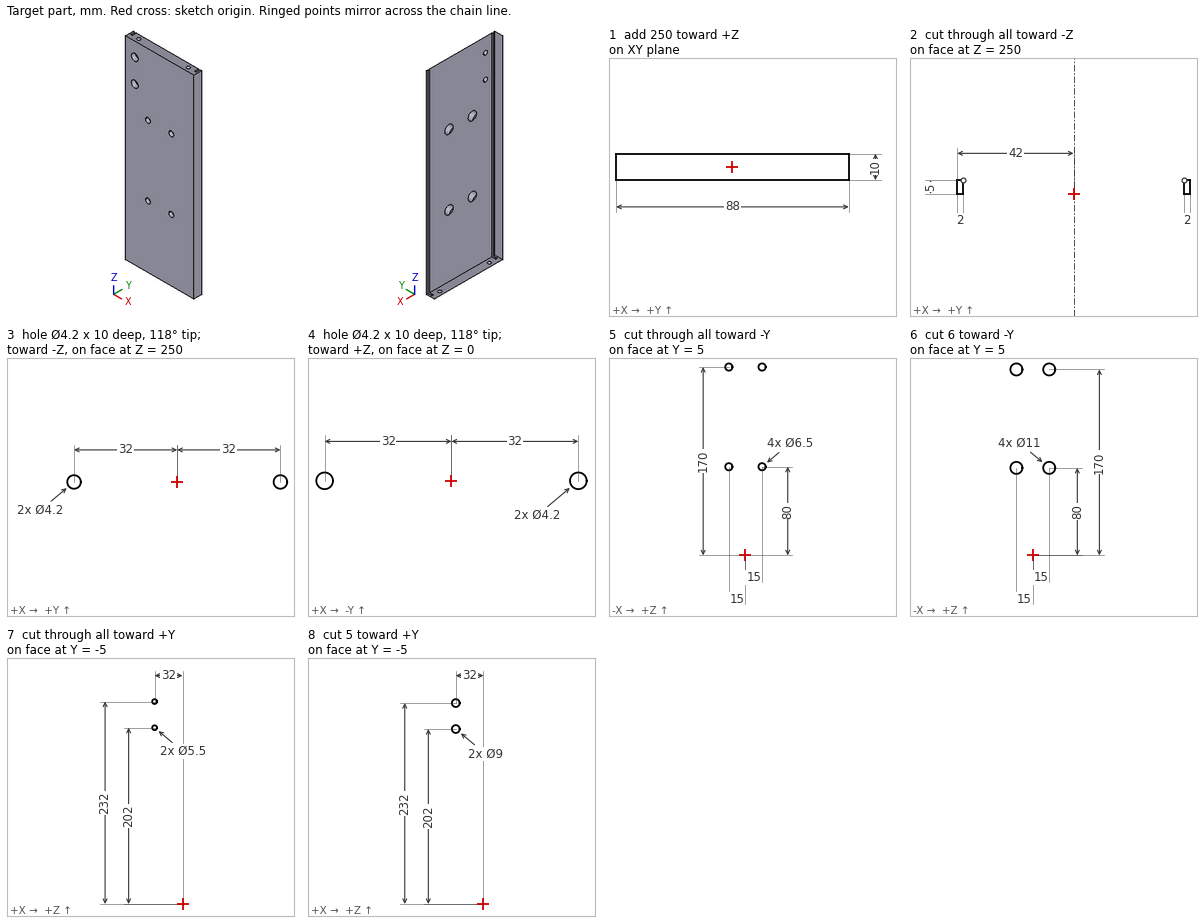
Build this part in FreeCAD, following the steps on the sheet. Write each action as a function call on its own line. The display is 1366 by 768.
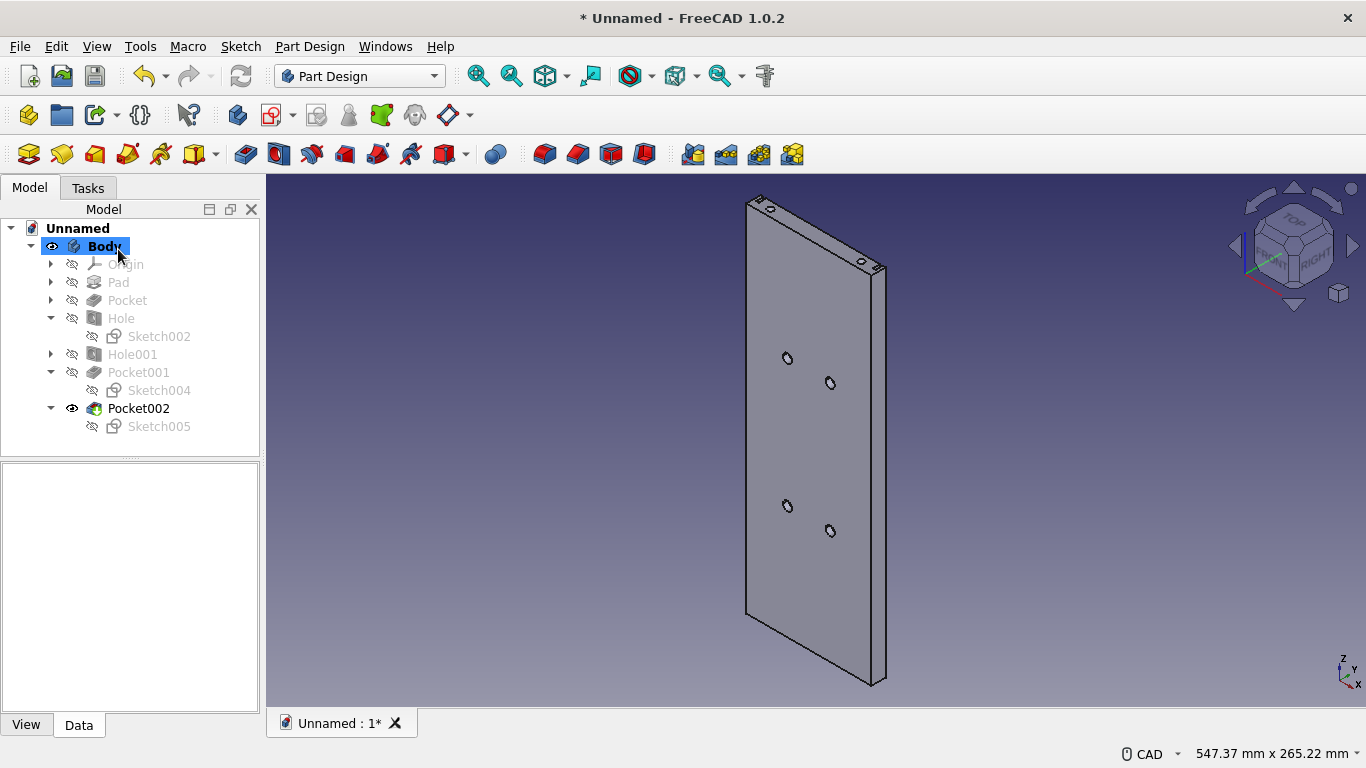
click(809, 444)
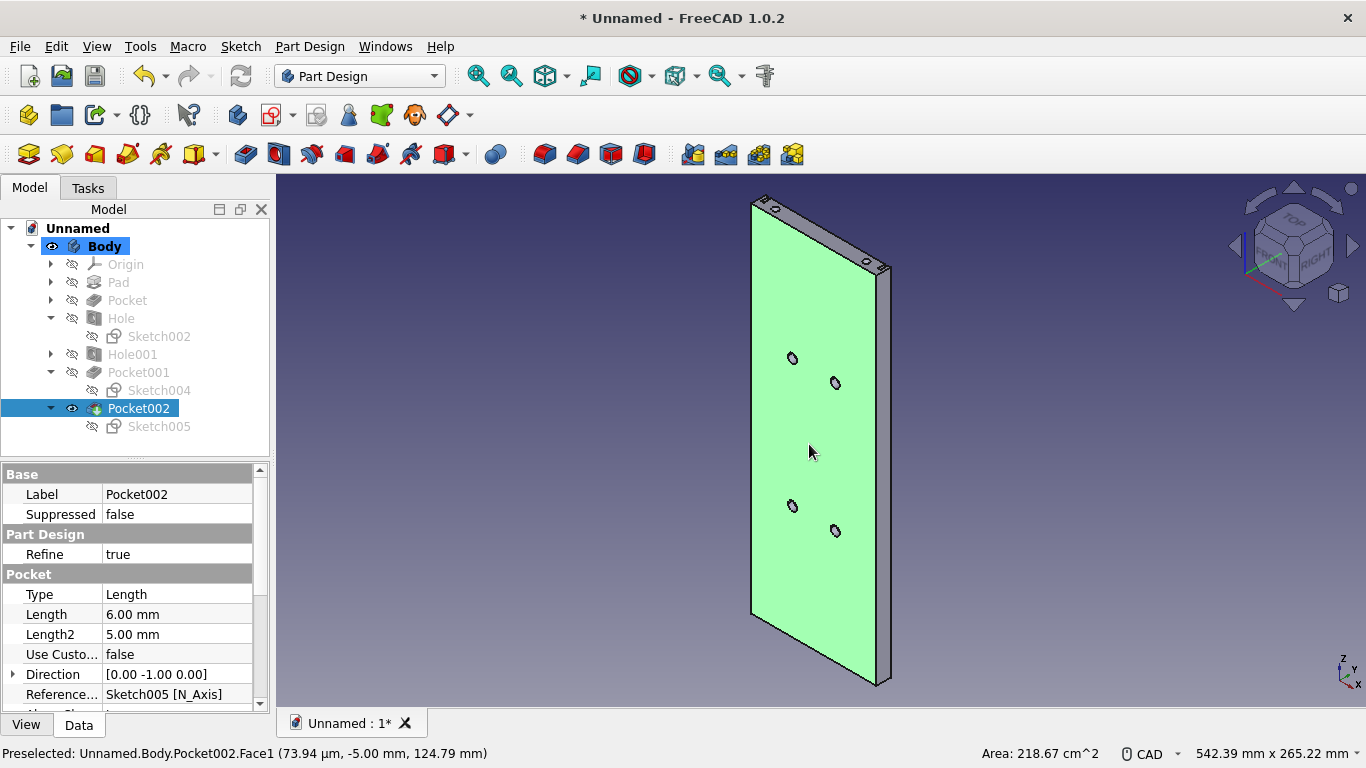
click(270, 116)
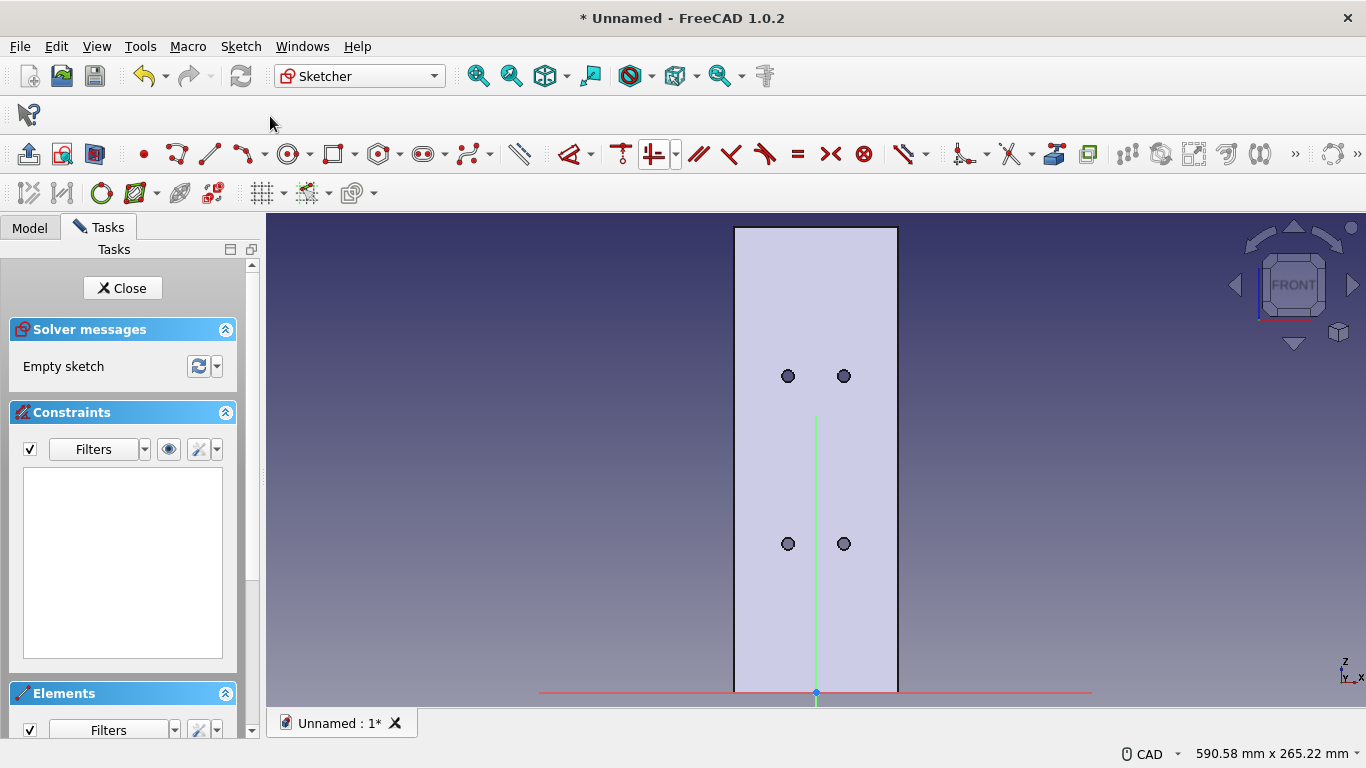
scroll(759, 245, up, 8)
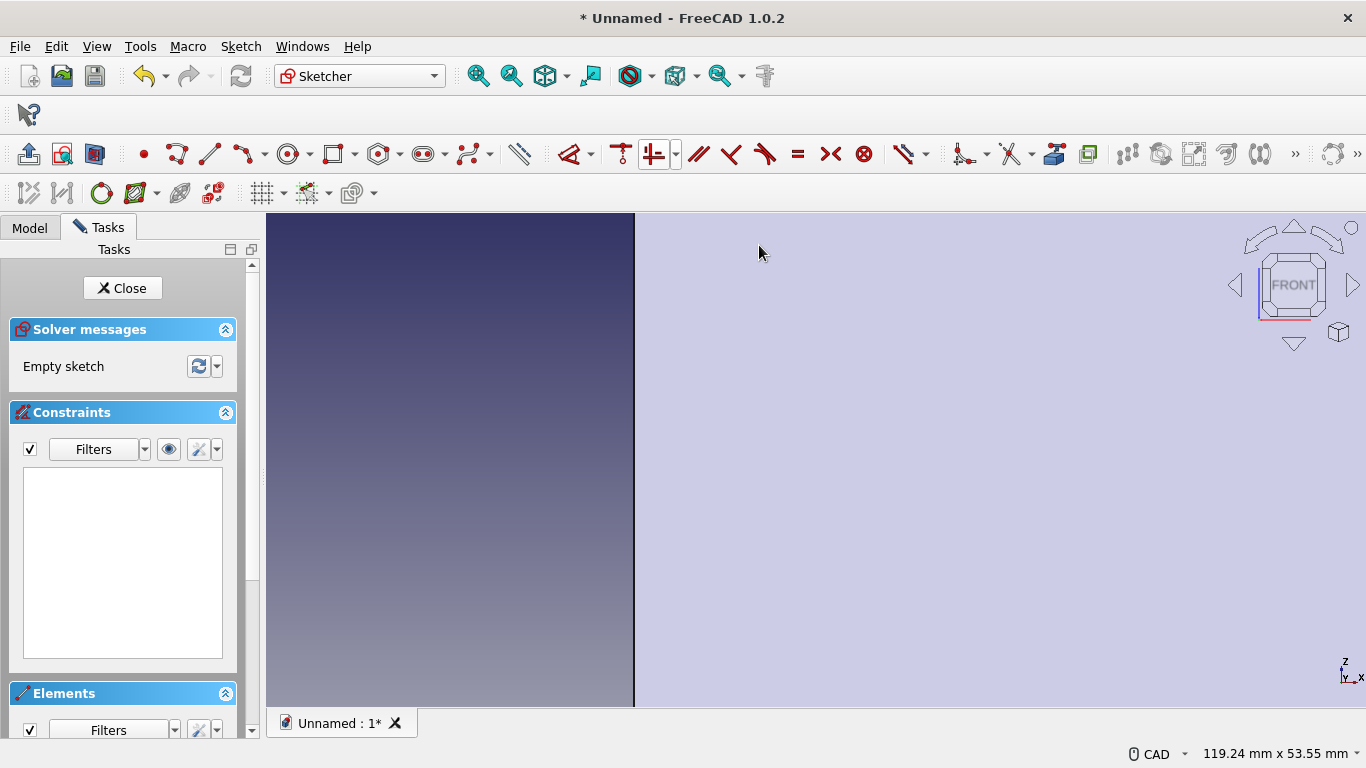
click(288, 154)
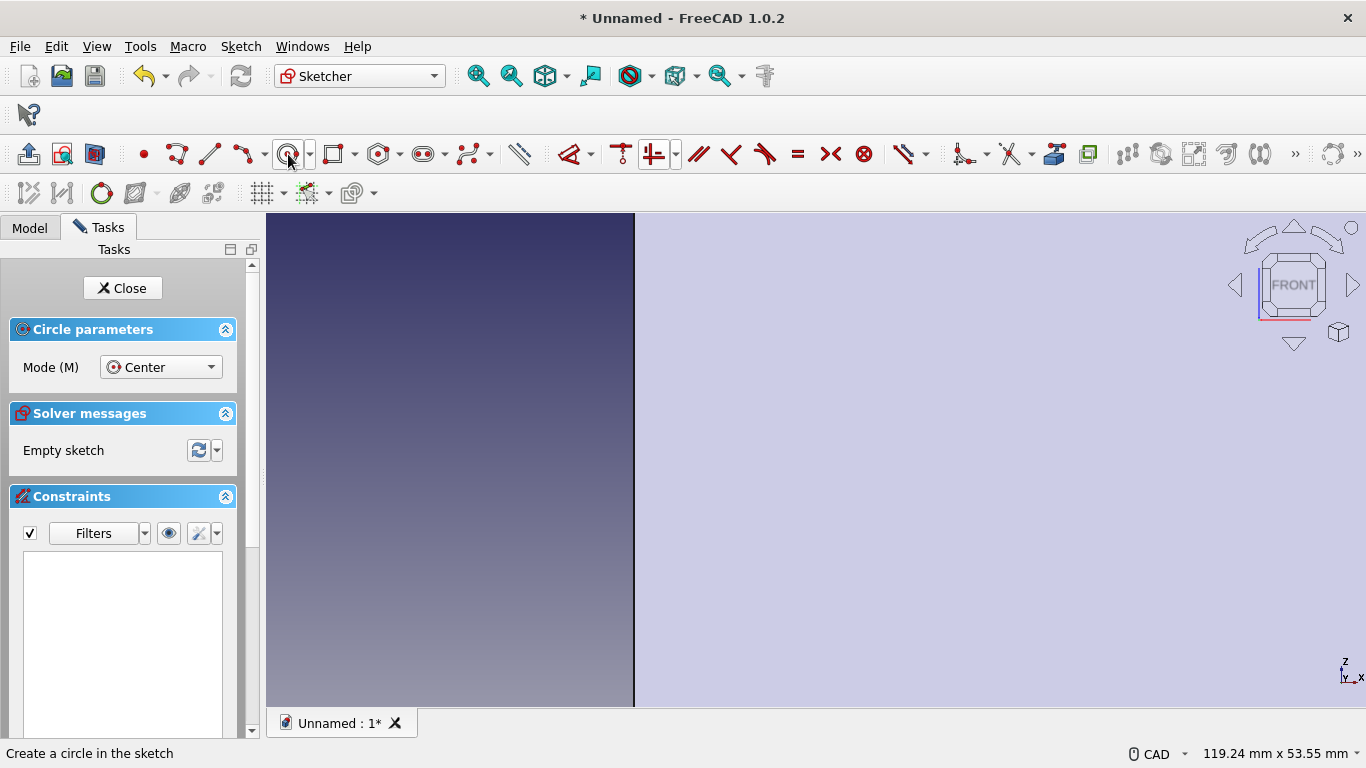
click(744, 323)
move(762, 305)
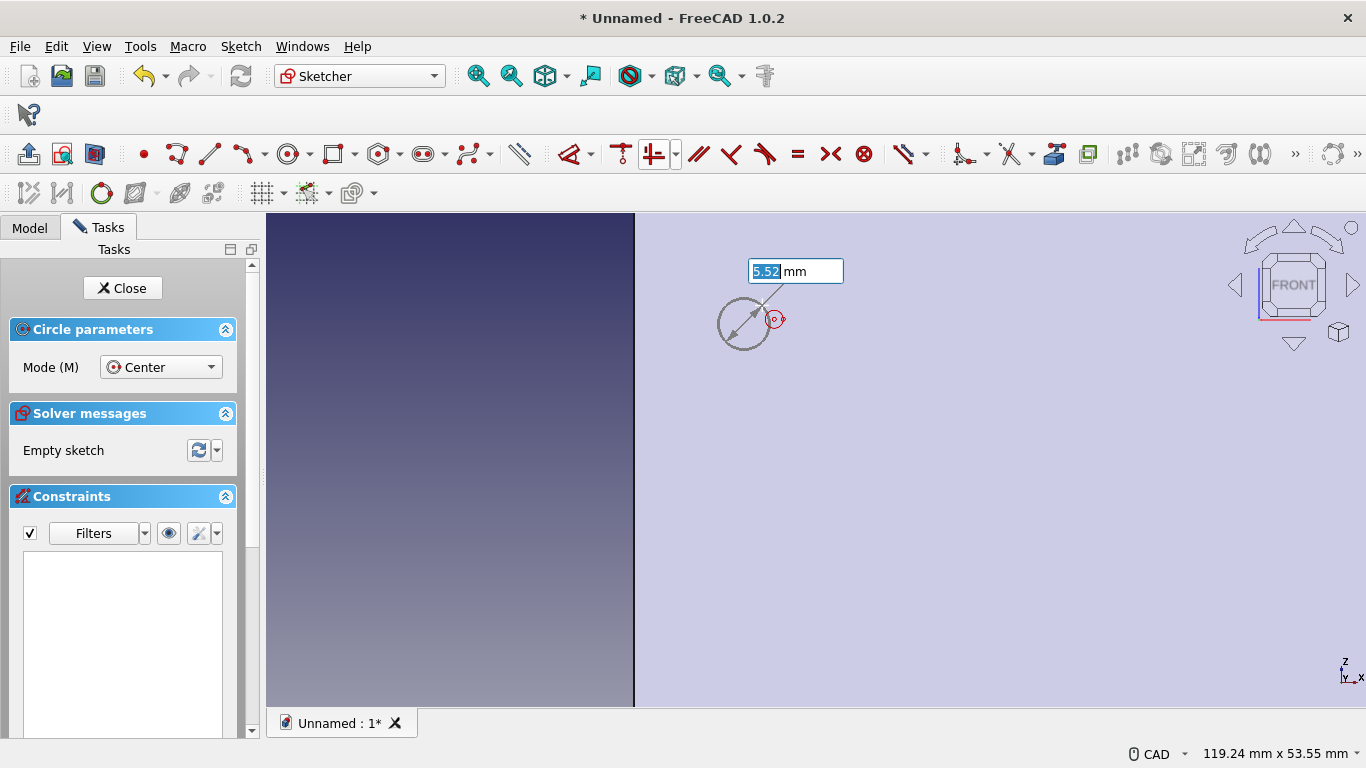
text(5.5)
key(Return)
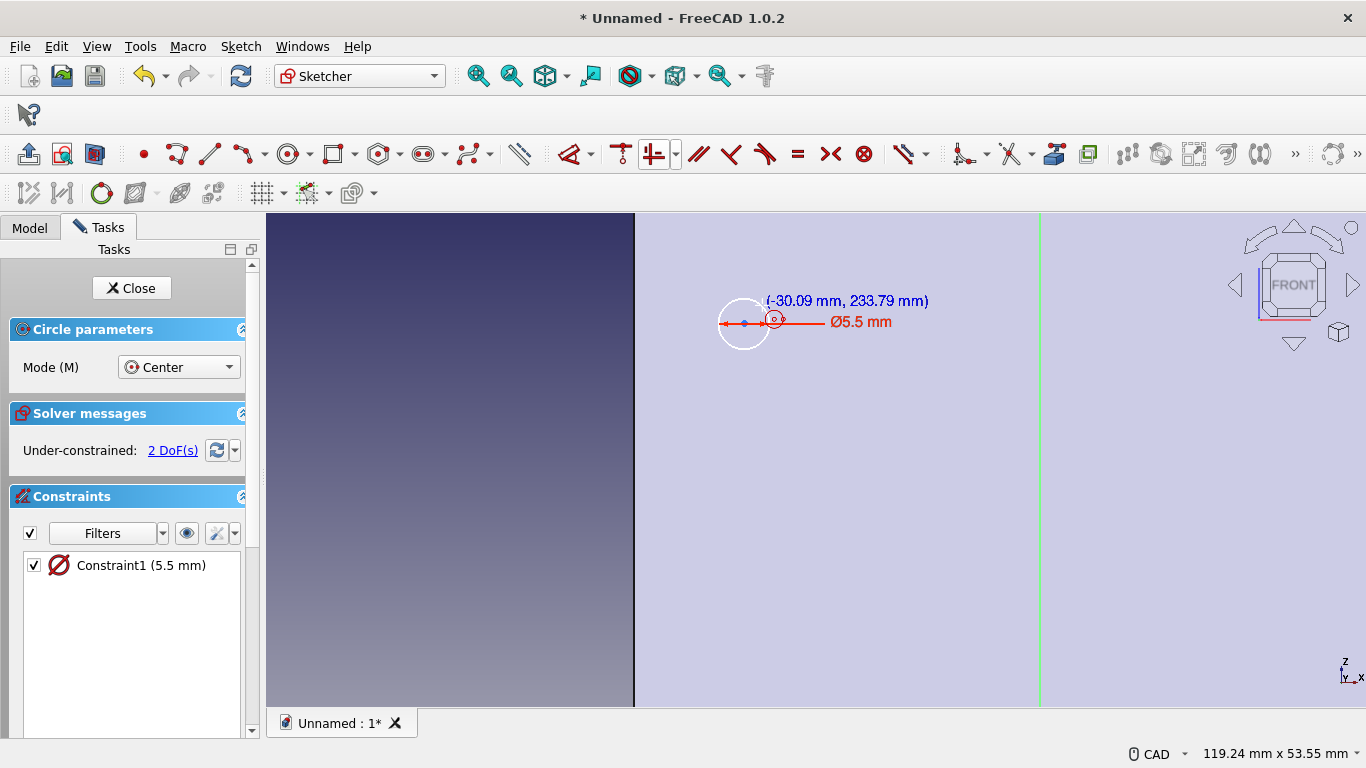
click(744, 599)
move(762, 581)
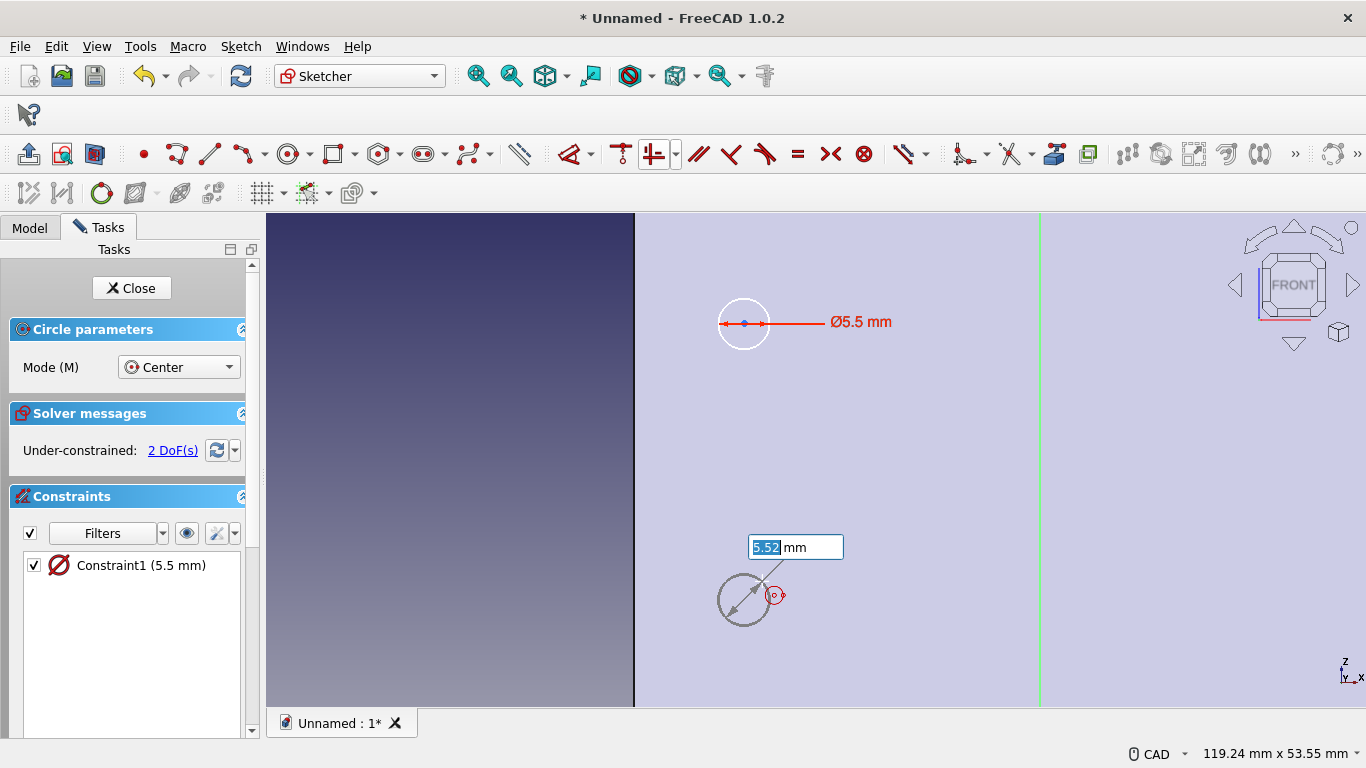
text(5.5)
key(Return)
key(Escape)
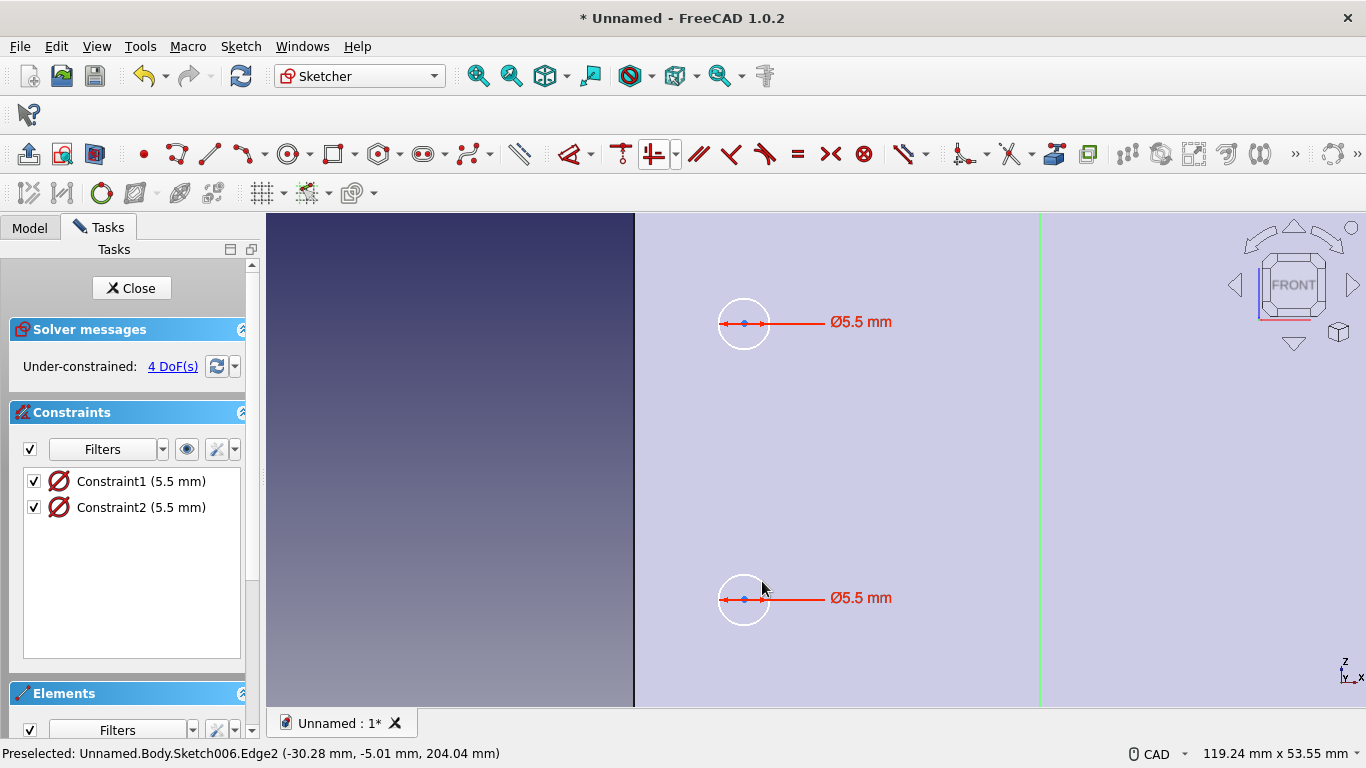
click(744, 324)